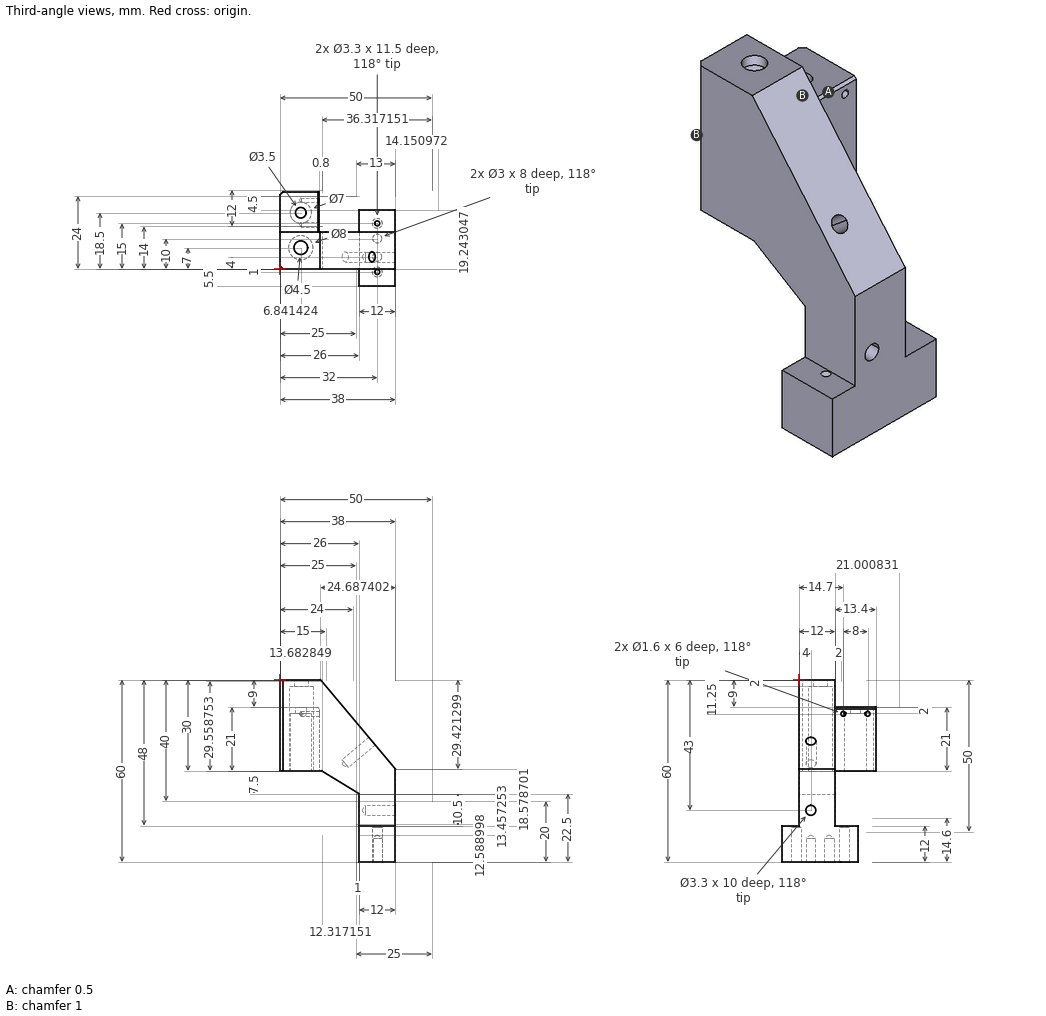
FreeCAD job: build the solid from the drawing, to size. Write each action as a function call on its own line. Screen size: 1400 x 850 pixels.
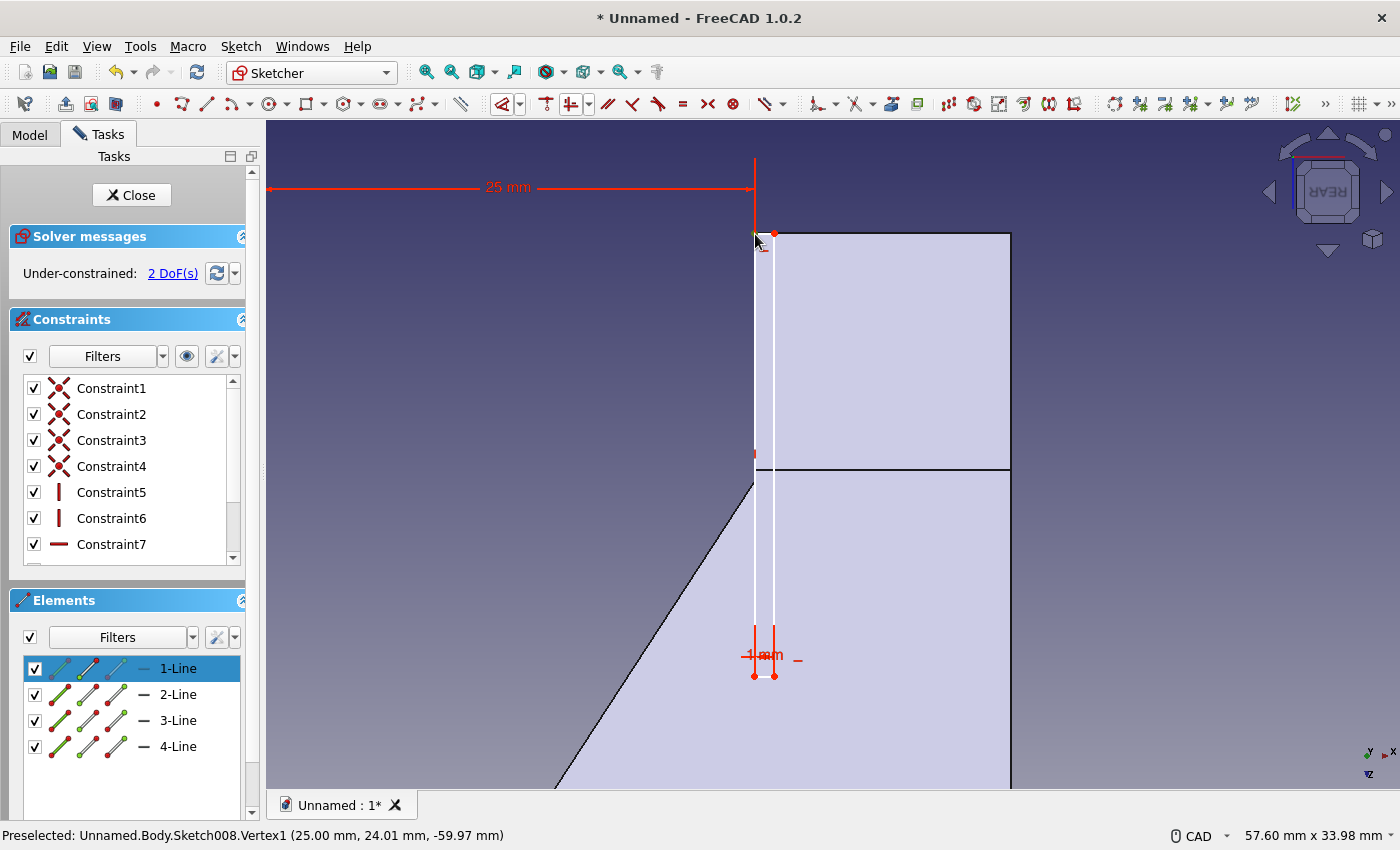
key(i)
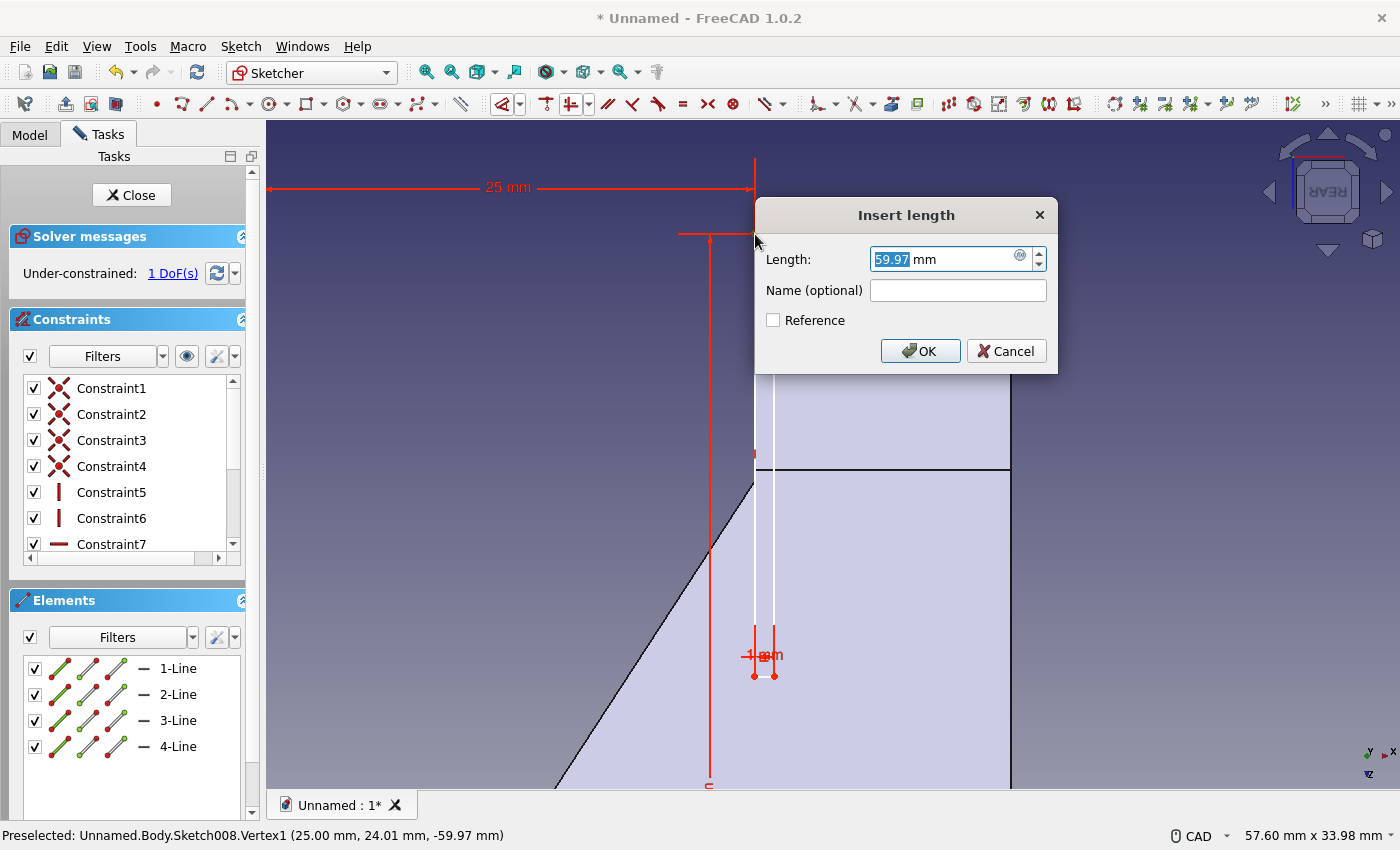
text(60)
key(Return)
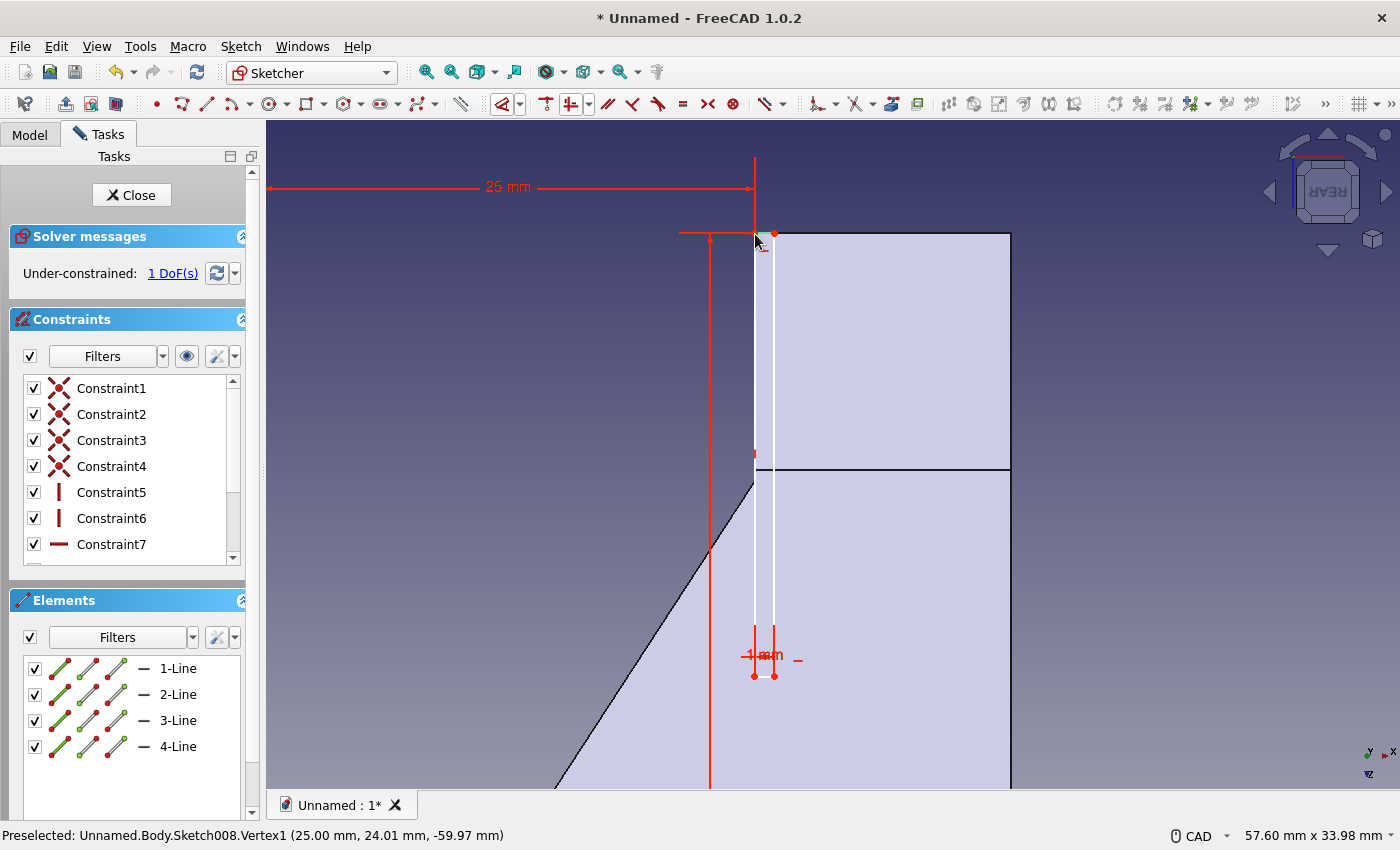
click(755, 366)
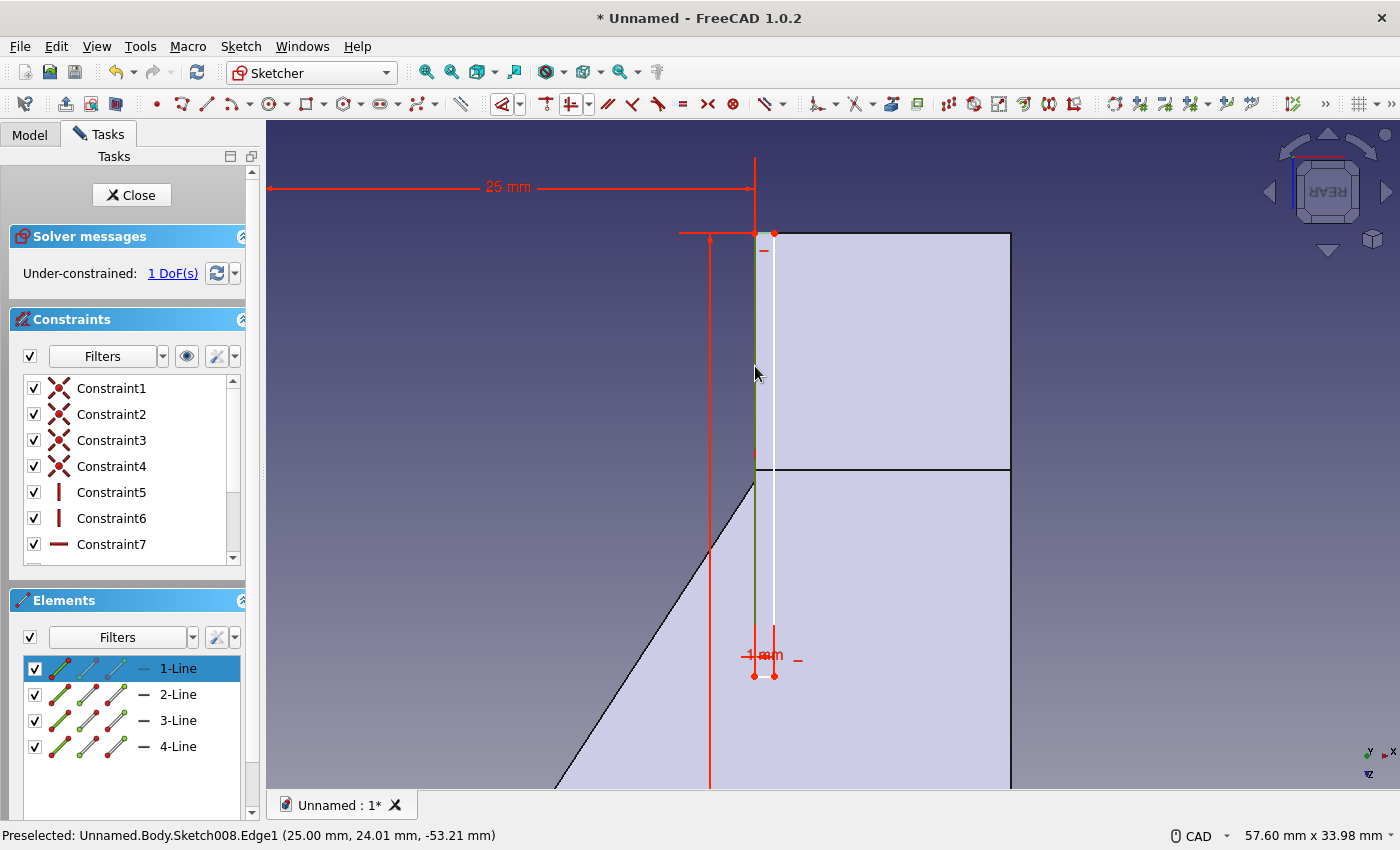
key(i)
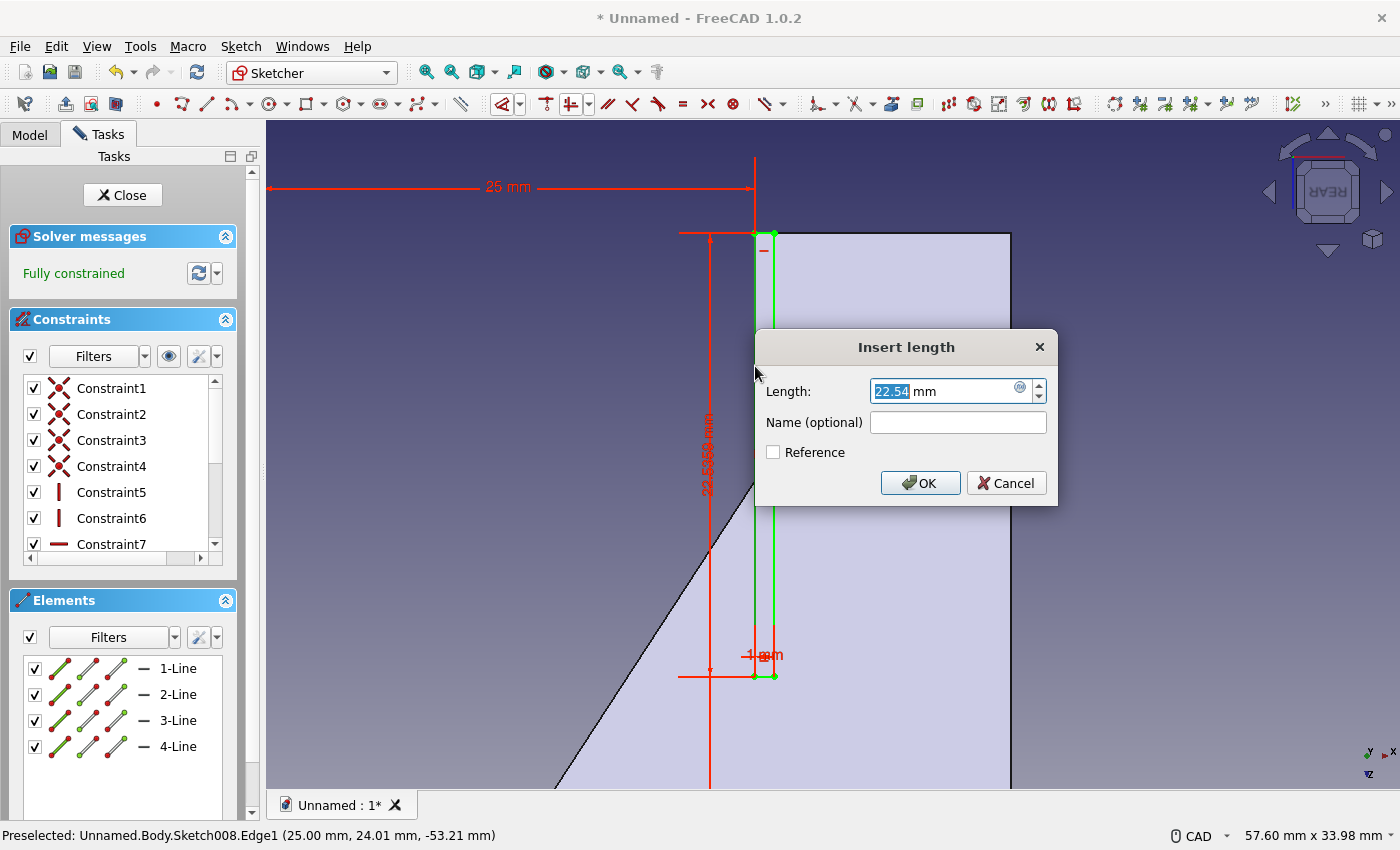
text(22.5)
key(Return)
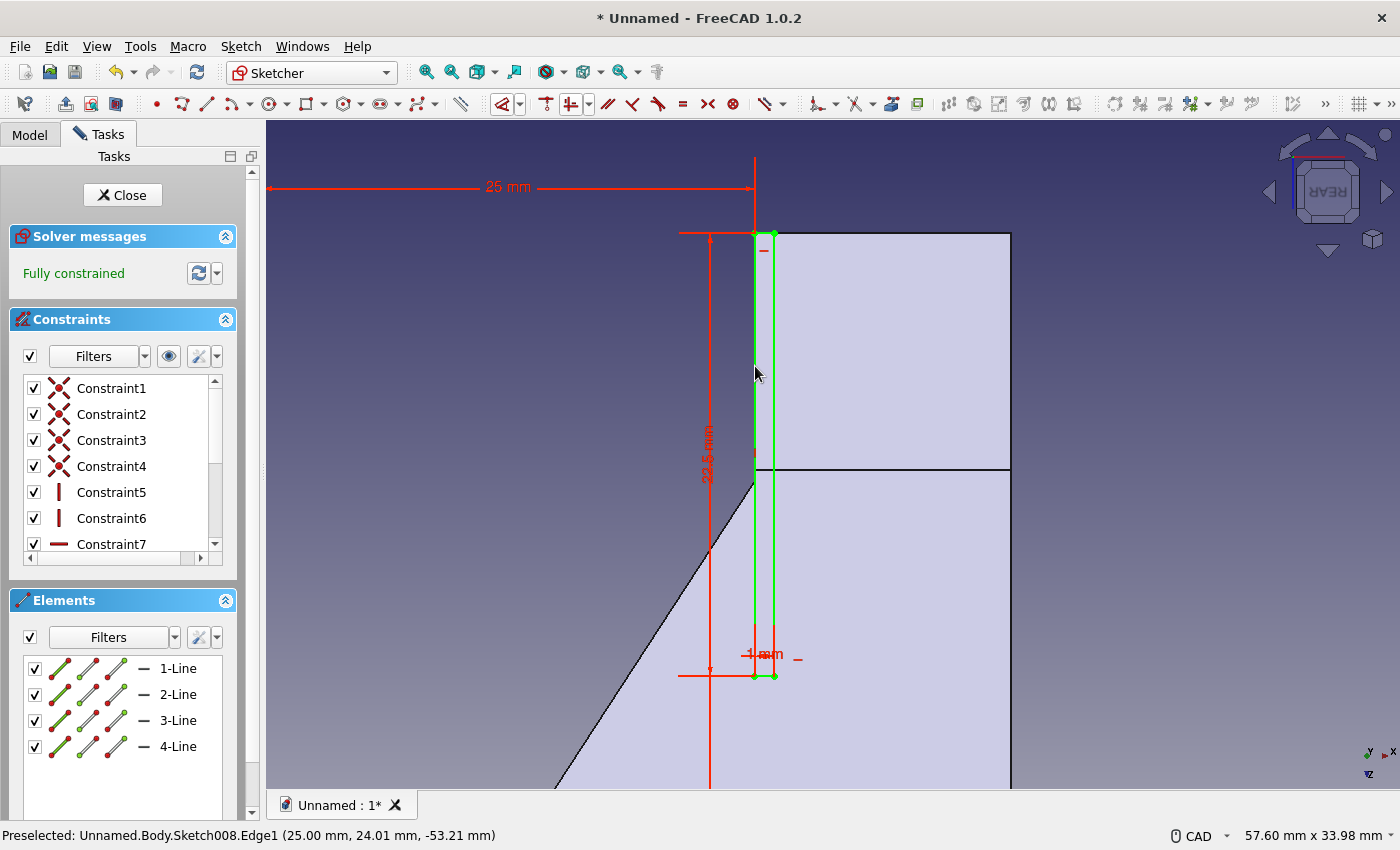
click(123, 195)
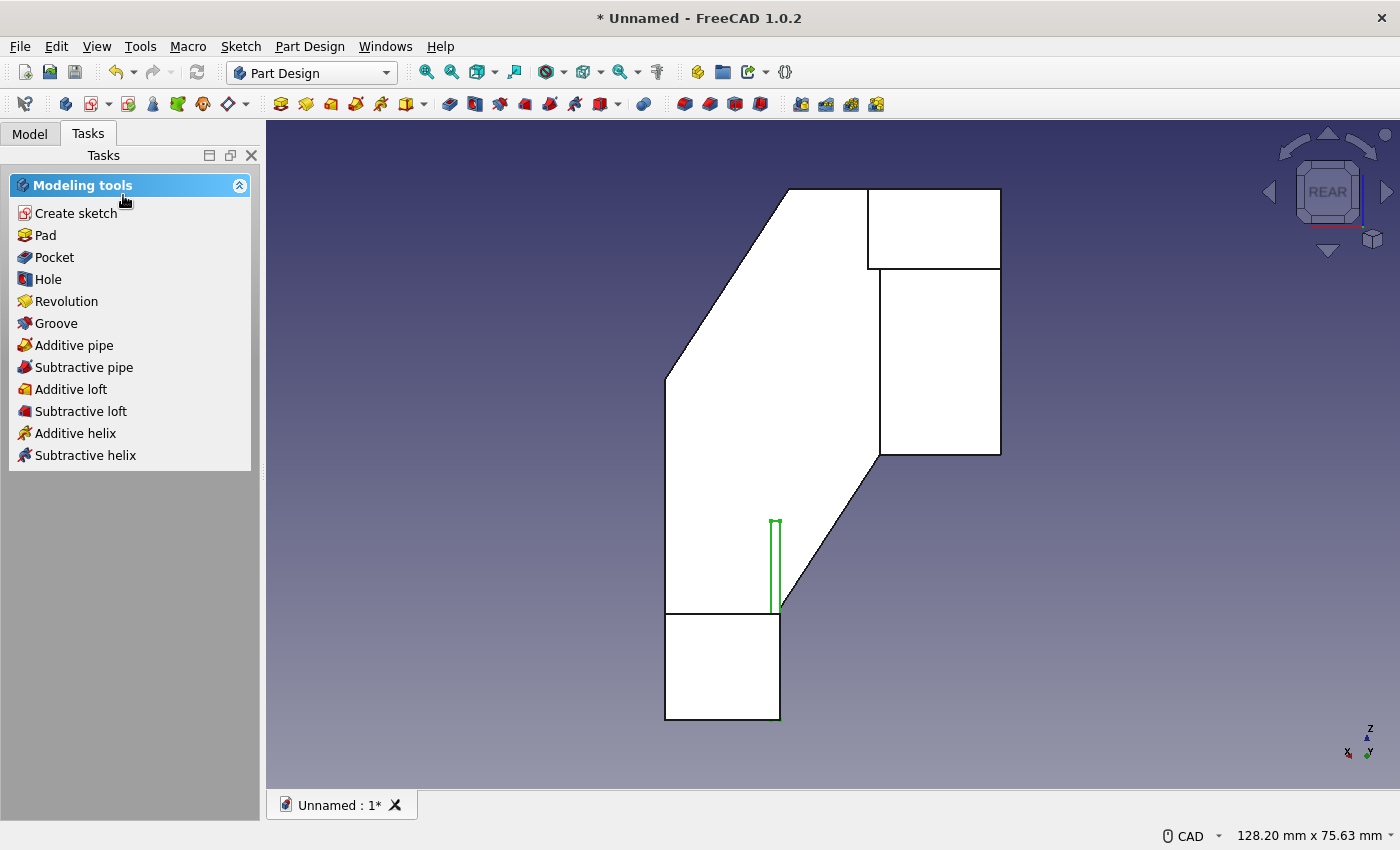
click(450, 104)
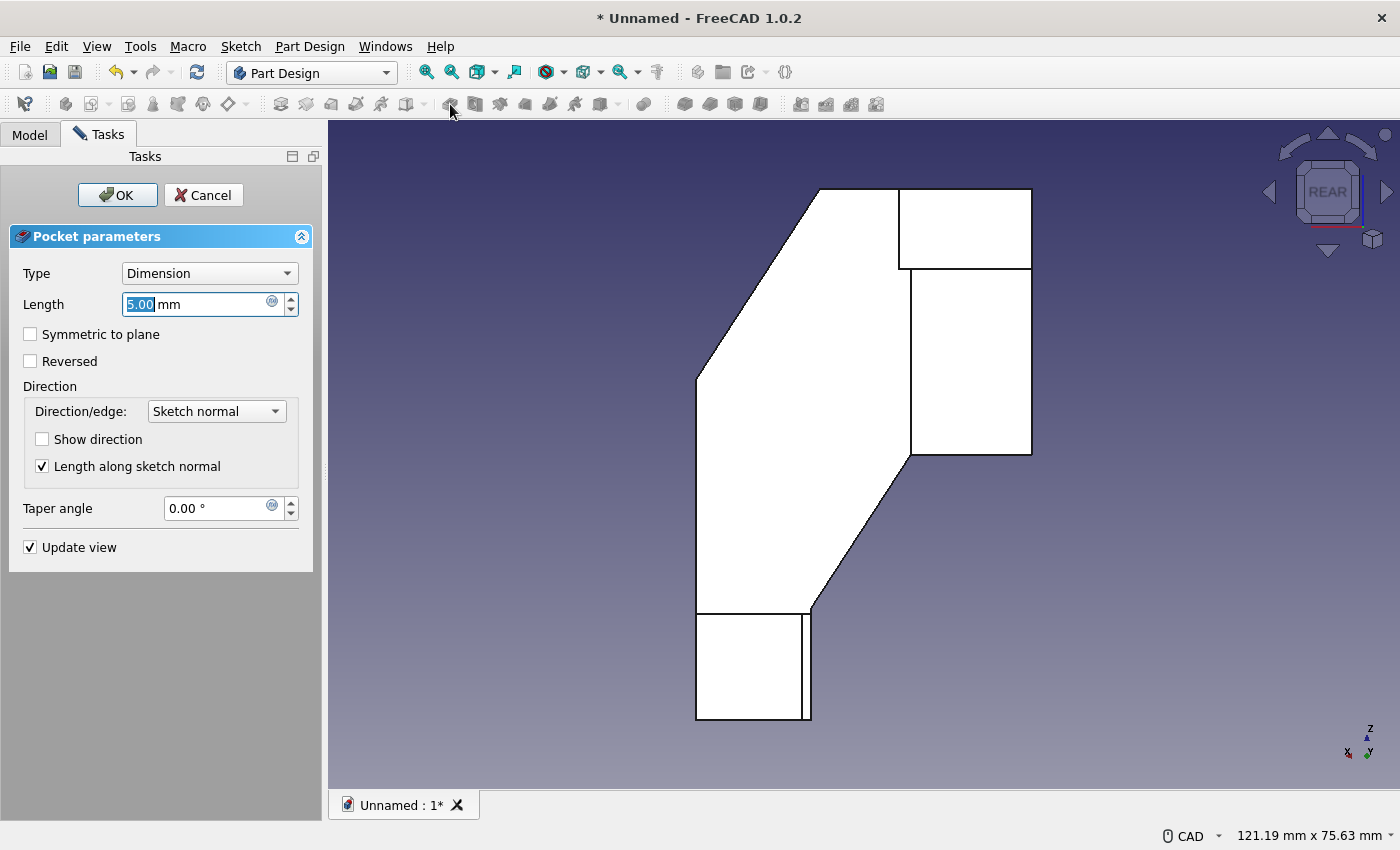
click(210, 274)